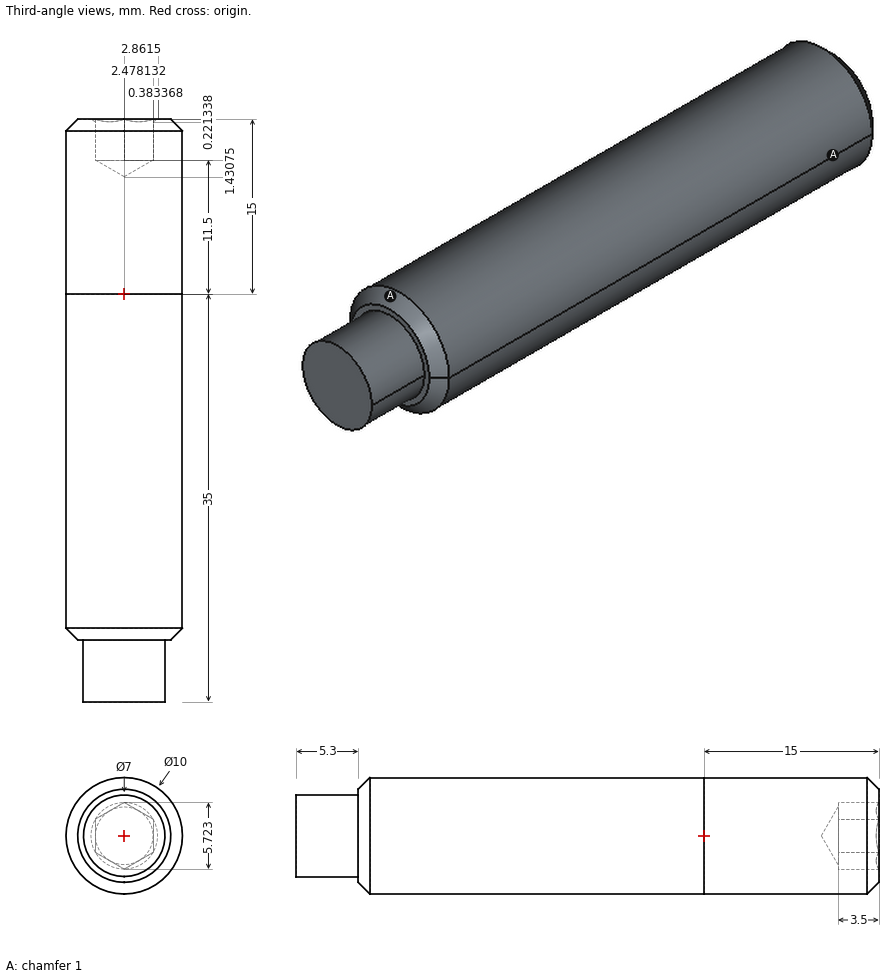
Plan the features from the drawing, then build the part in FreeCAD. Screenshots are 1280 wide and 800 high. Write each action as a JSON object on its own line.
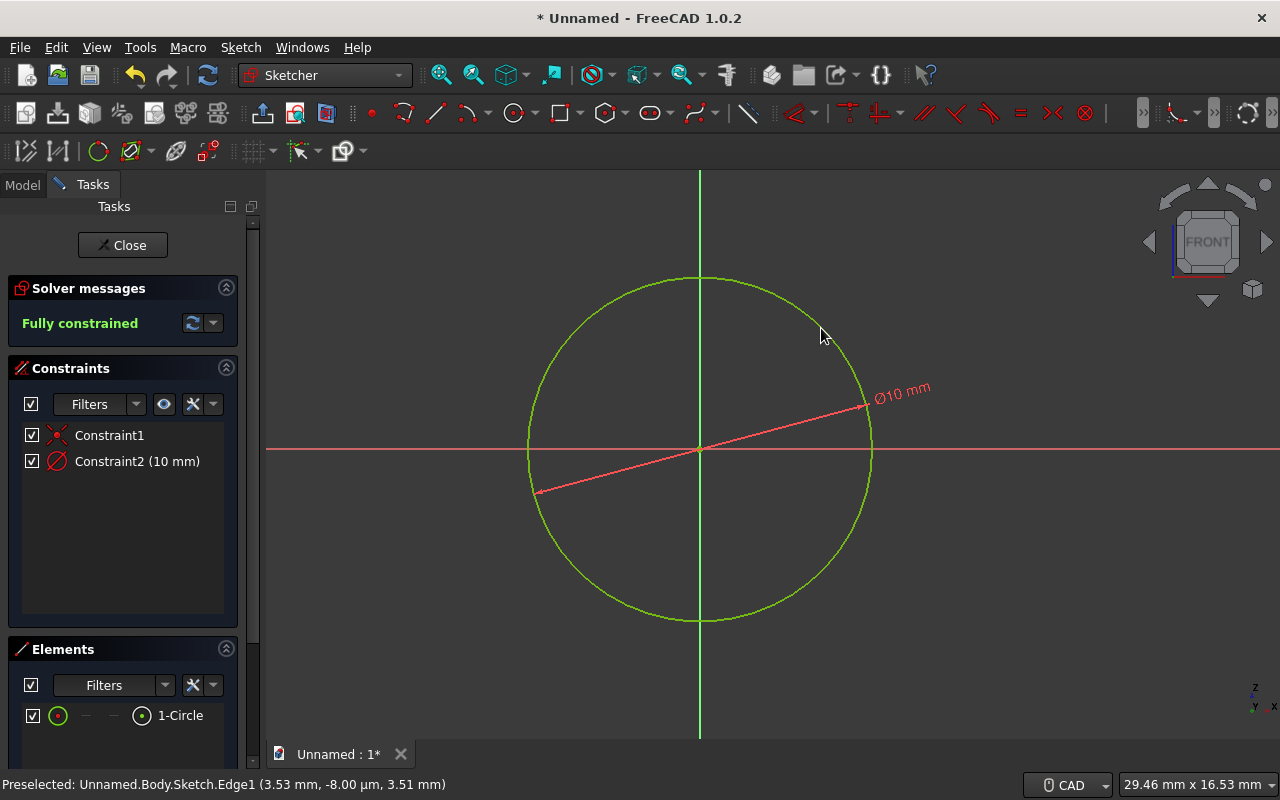
{"action": "left_click", "coordinate": [123, 245]}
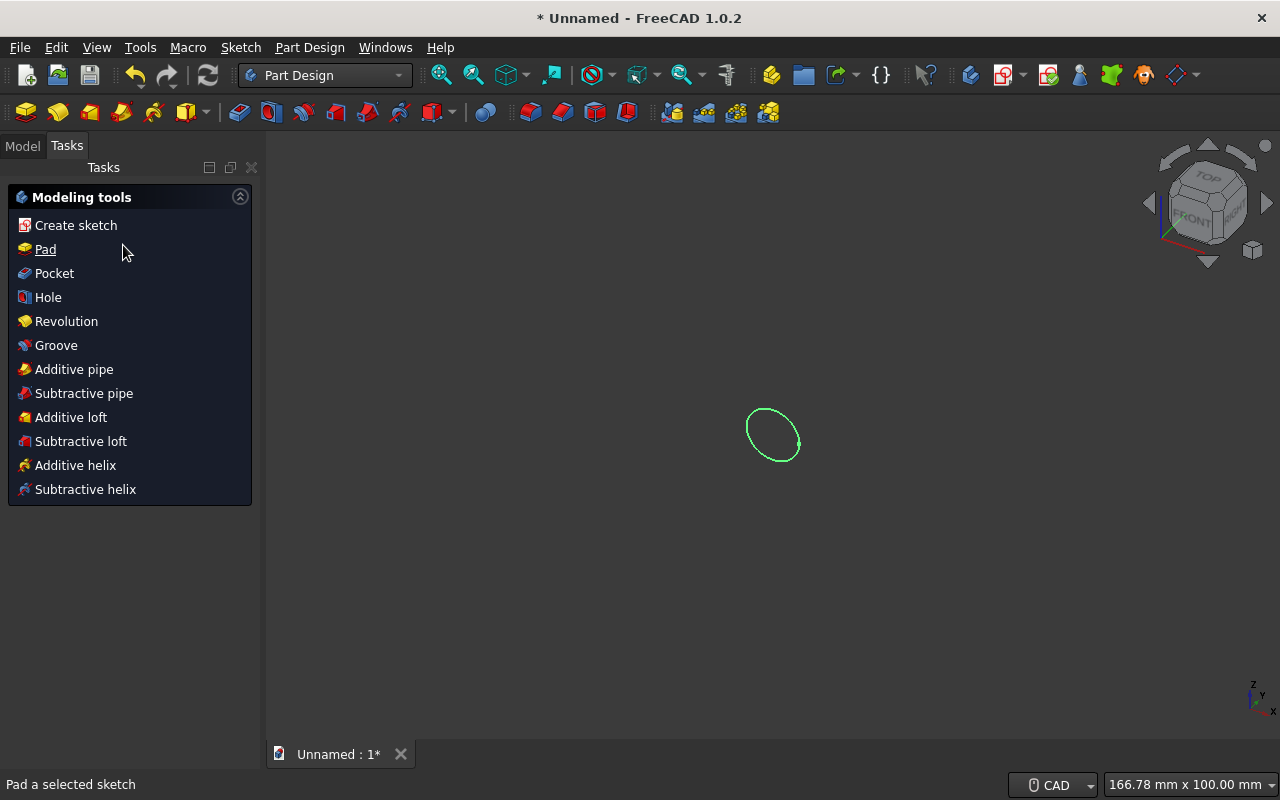
{"action": "left_click", "coordinate": [26, 112]}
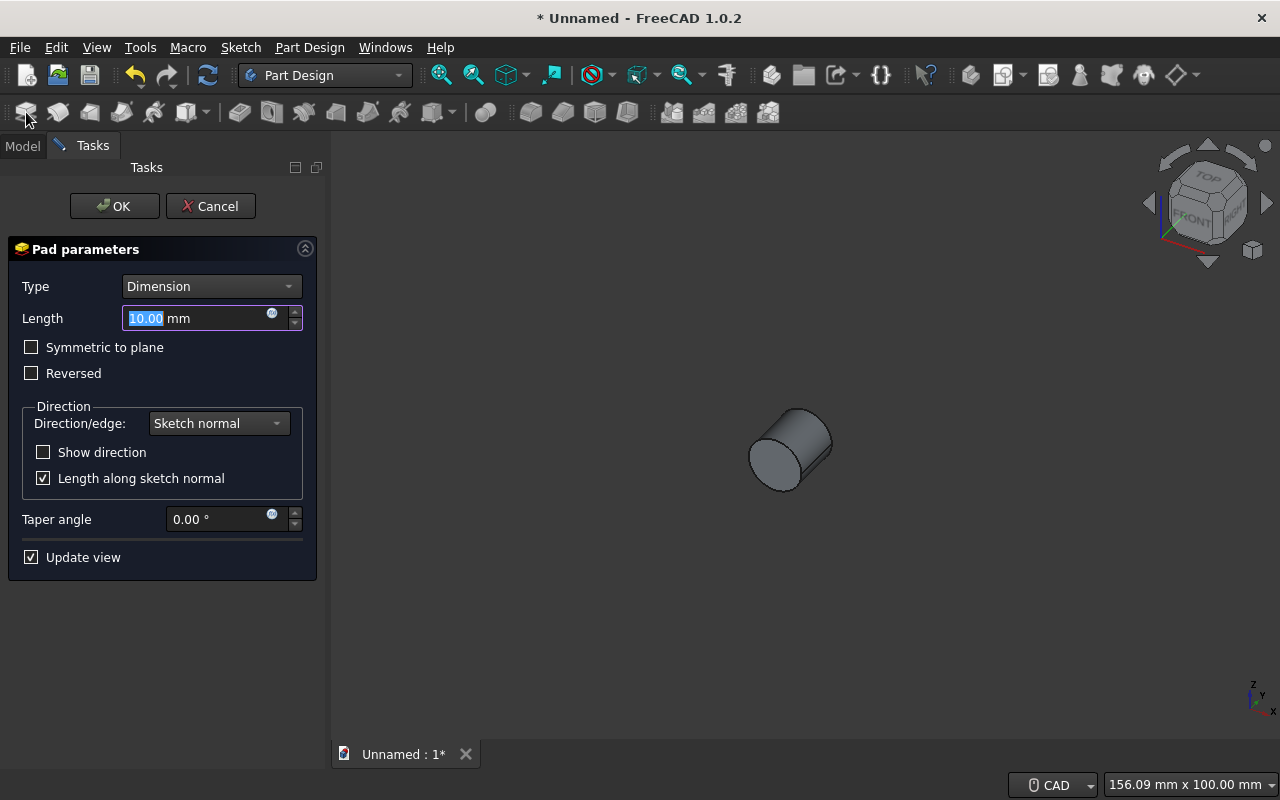
{"action": "type", "text": "15"}
{"action": "key", "text": "Tab"}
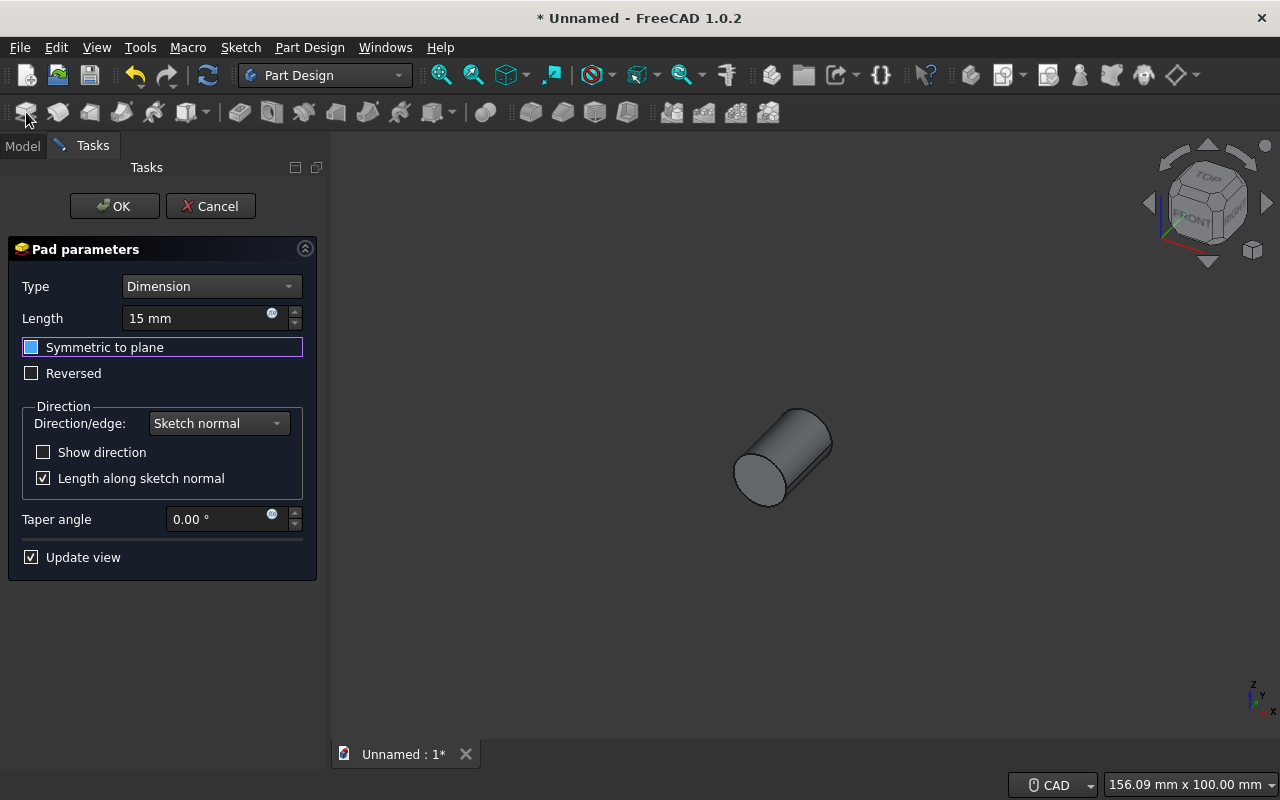
{"action": "left_click", "coordinate": [30, 373]}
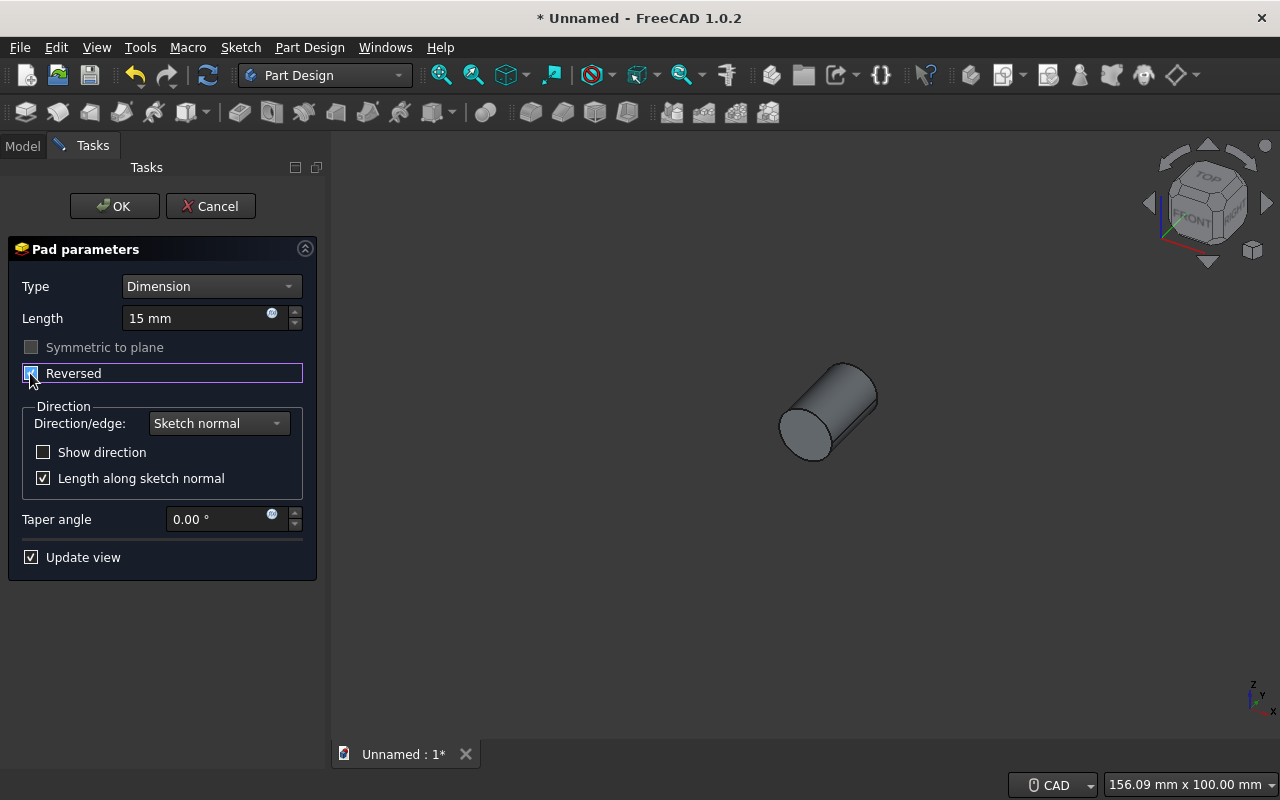
{"action": "left_click", "coordinate": [115, 206]}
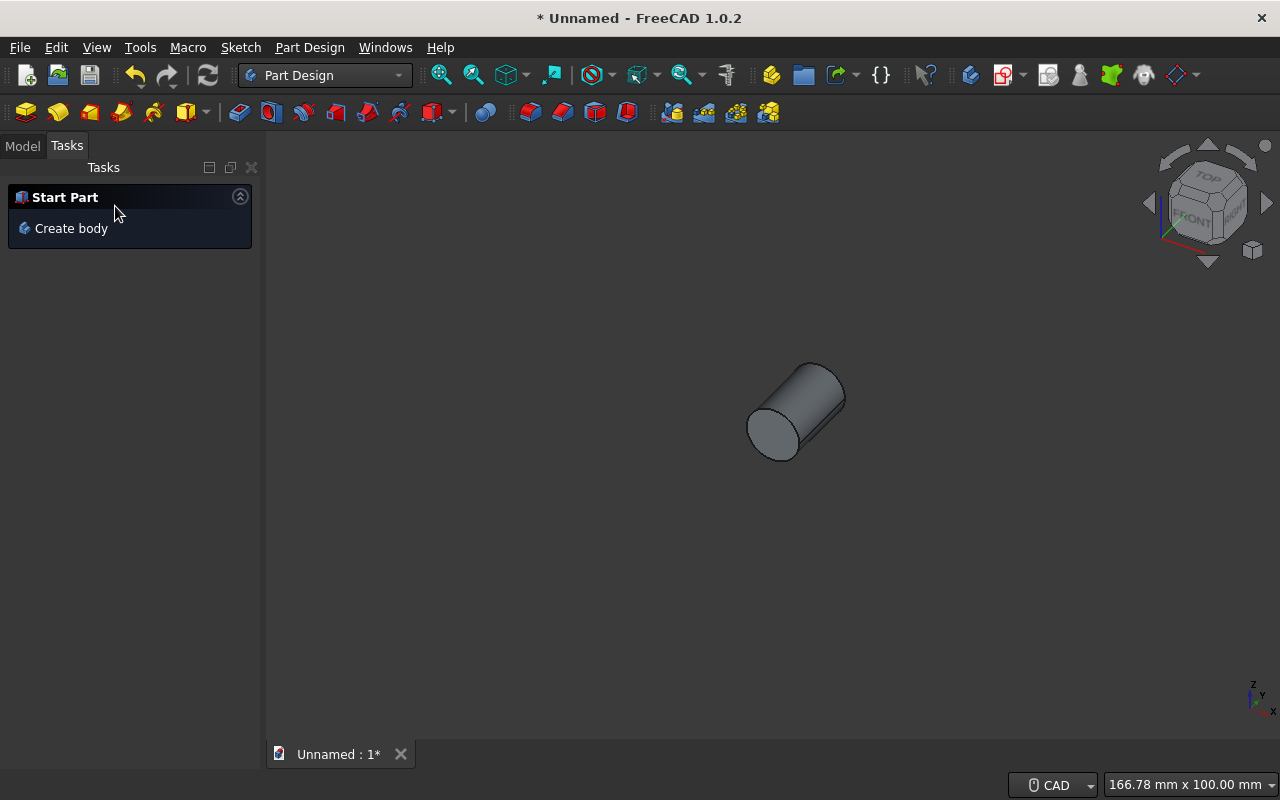
{"action": "left_click", "coordinate": [442, 76]}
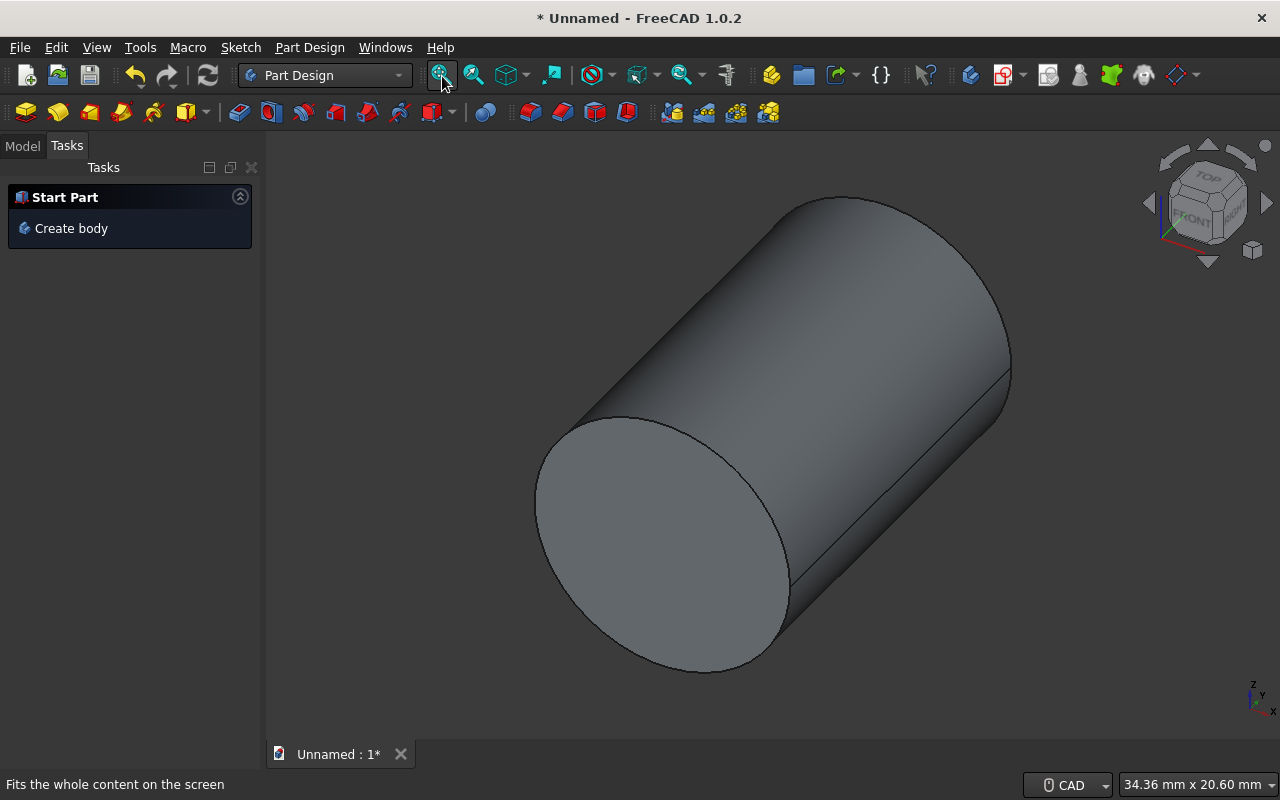
{"action": "left_click", "coordinate": [23, 145]}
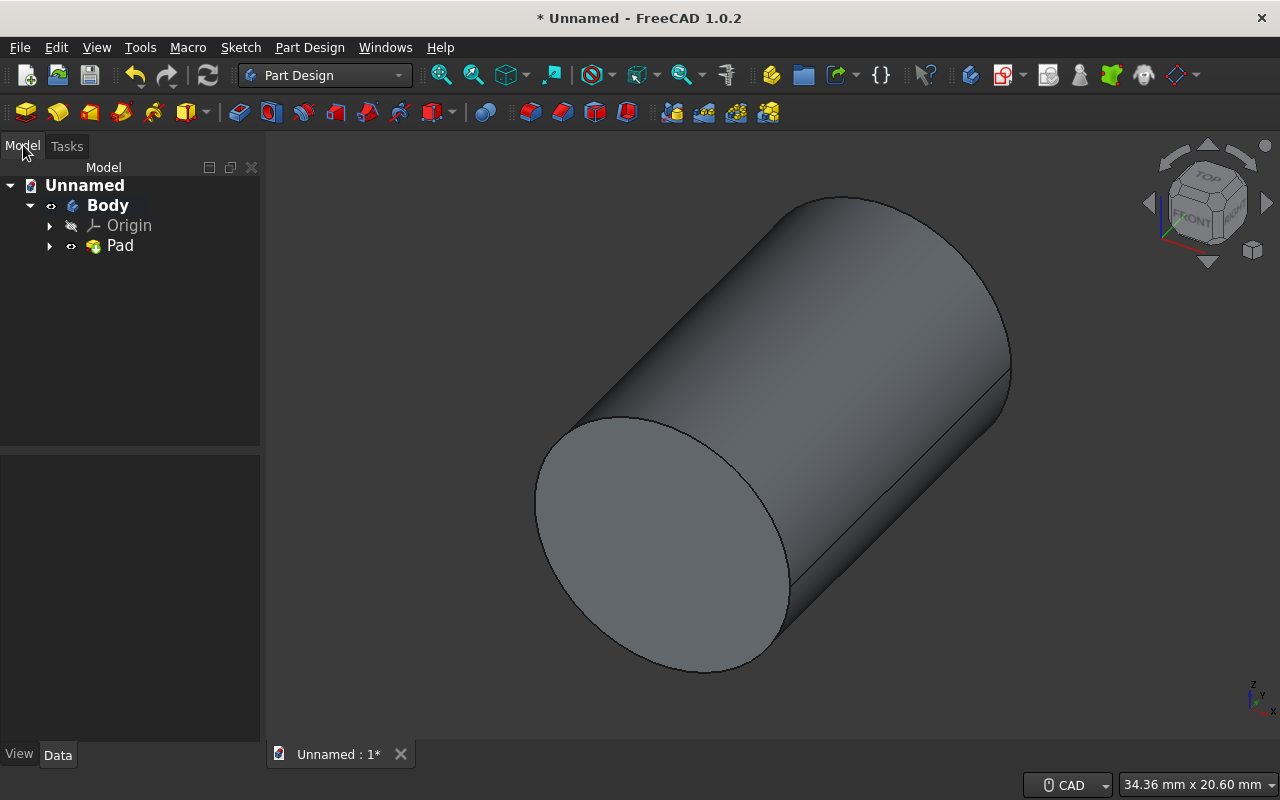
{"action": "left_click", "coordinate": [50, 226]}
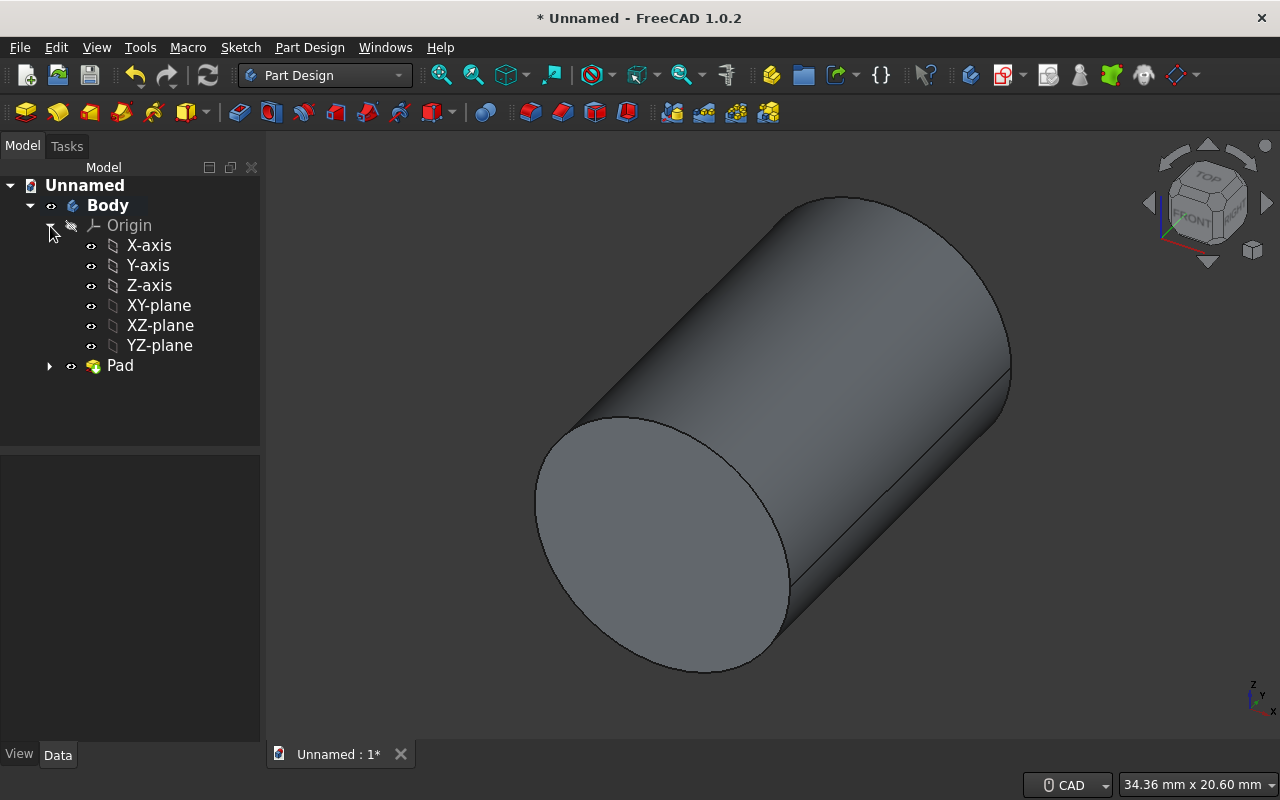
{"action": "left_click", "coordinate": [136, 326]}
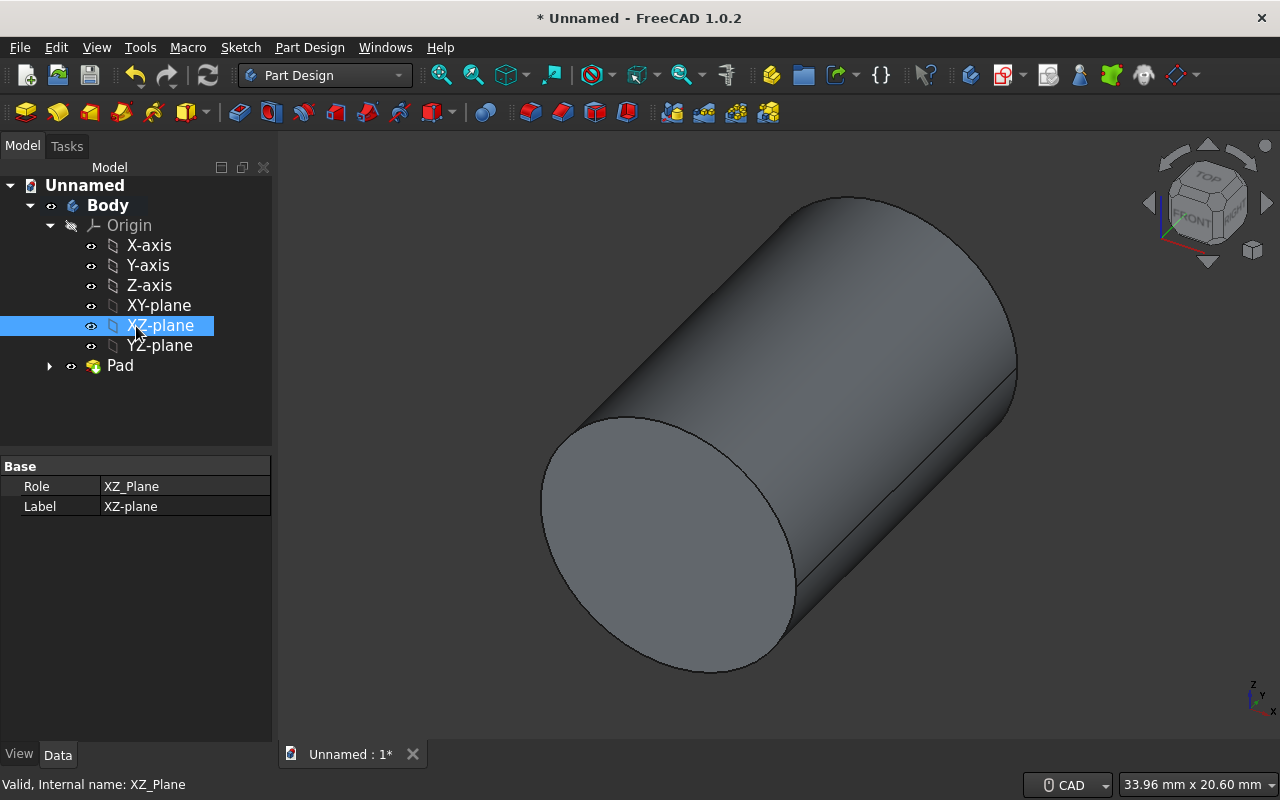
{"action": "left_click", "coordinate": [1176, 76]}